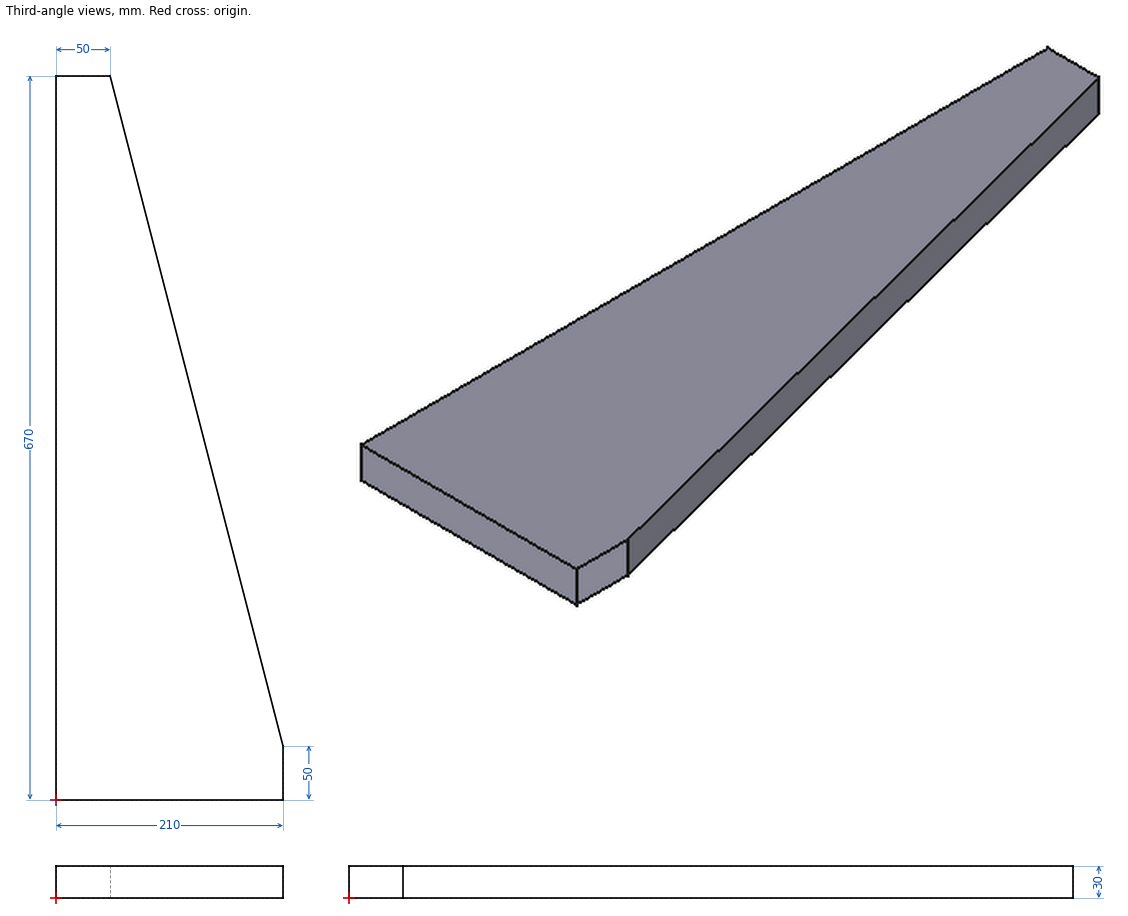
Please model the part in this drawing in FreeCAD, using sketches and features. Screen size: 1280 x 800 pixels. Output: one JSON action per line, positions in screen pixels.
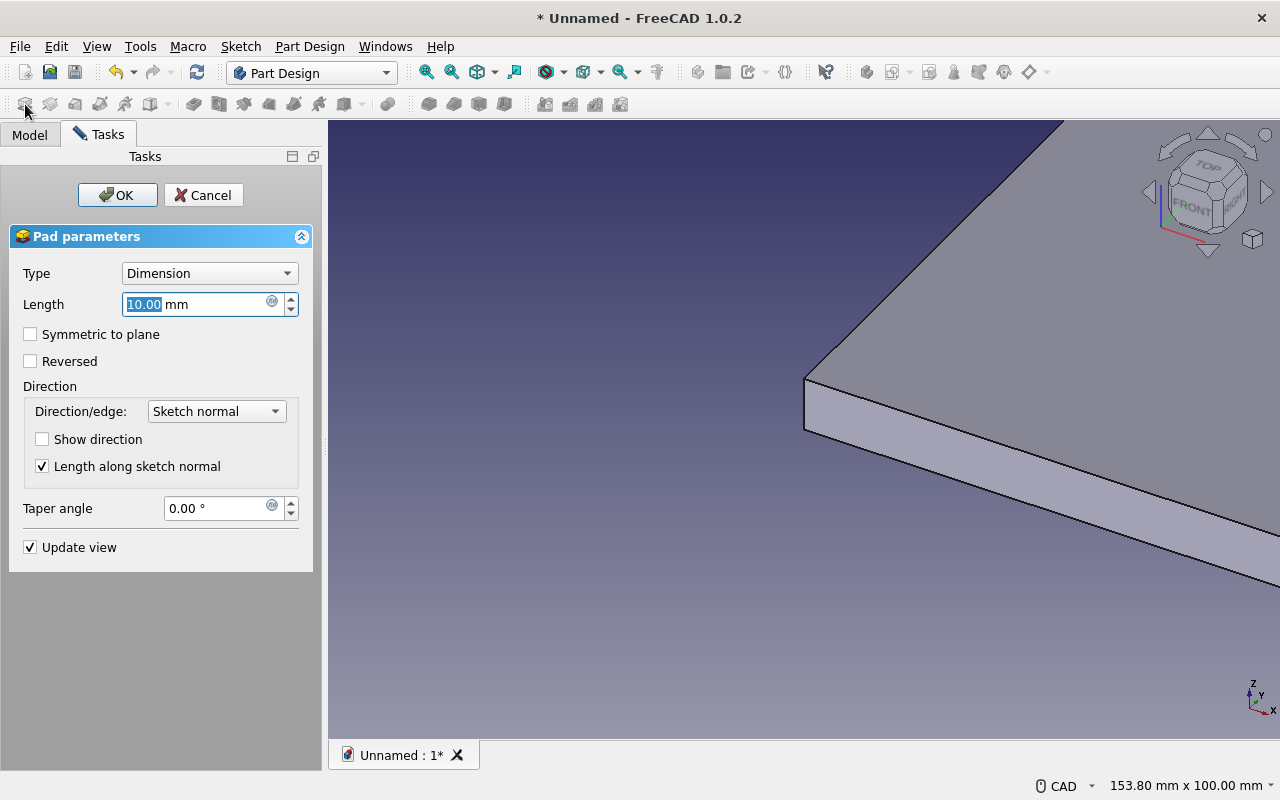
{"action": "type", "text": "30"}
{"action": "key", "text": "Tab"}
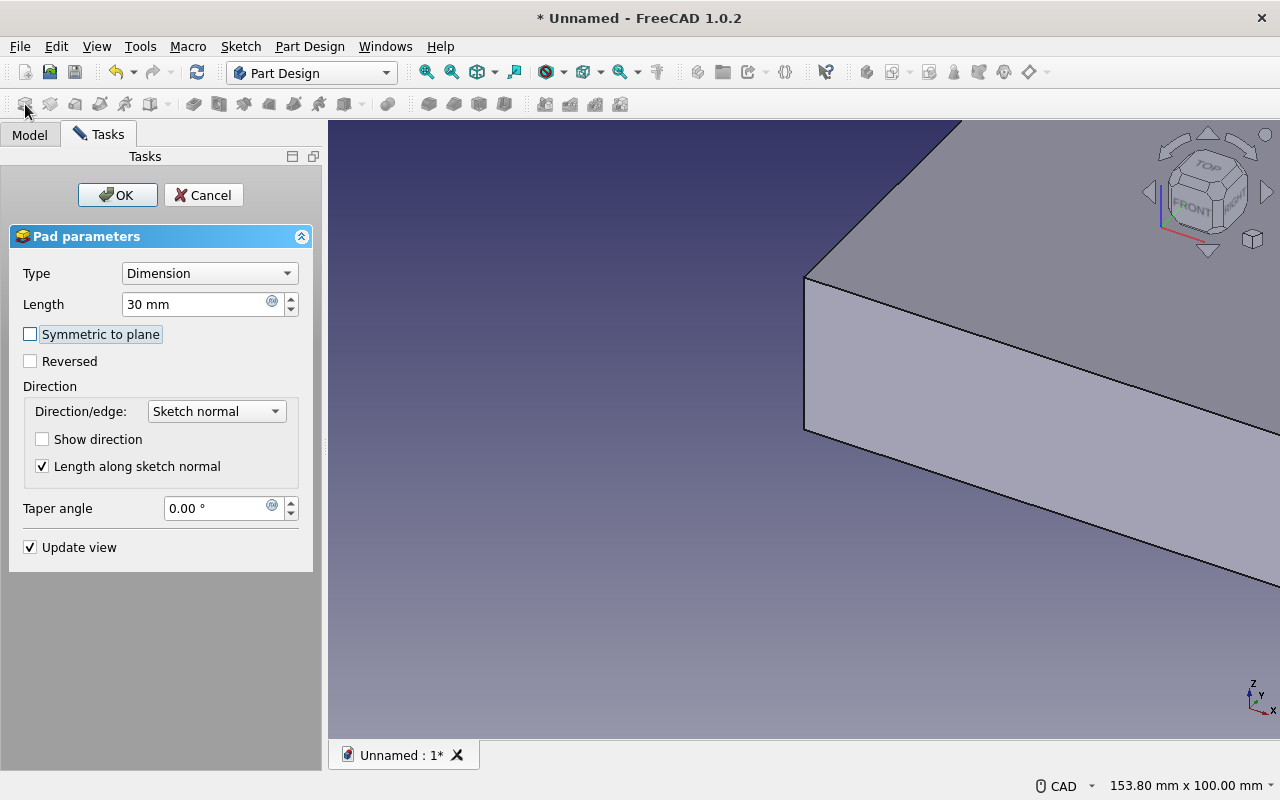
{"action": "left_click", "coordinate": [118, 195]}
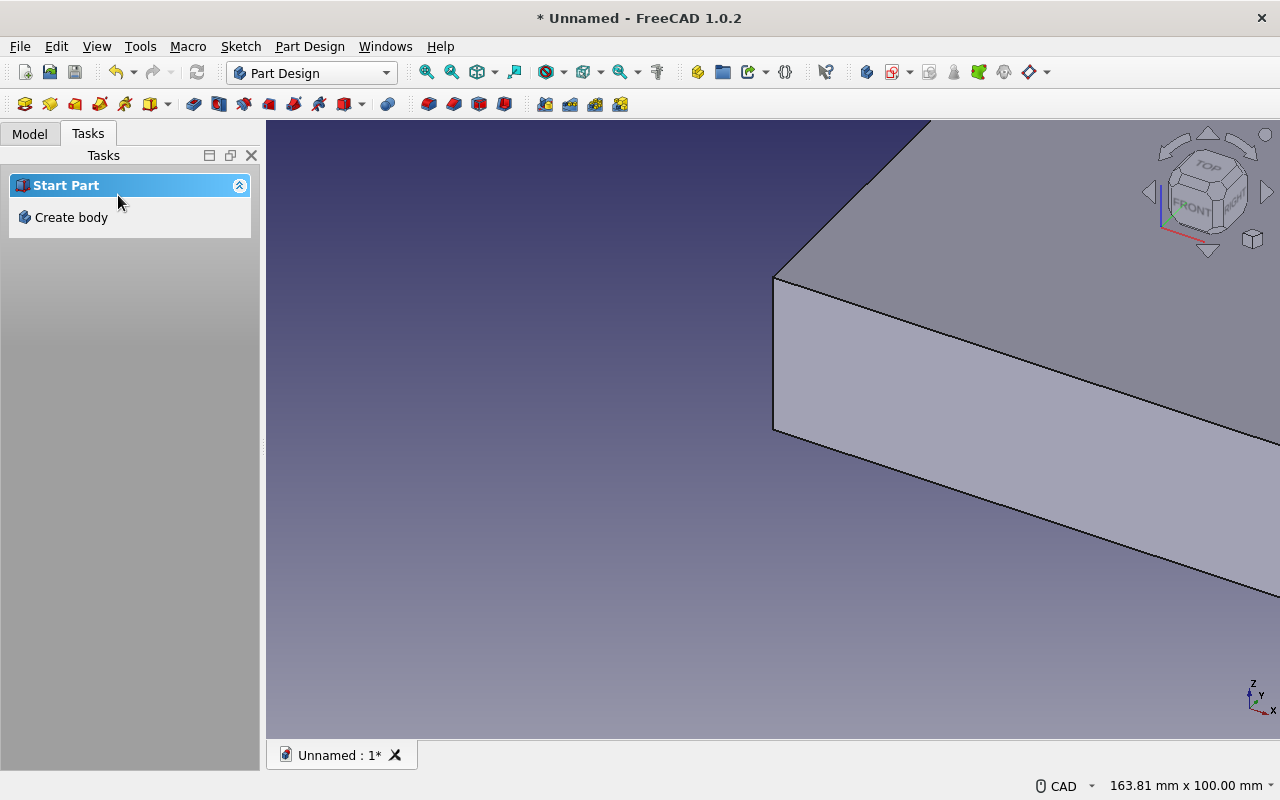
{"action": "key", "text": "0"}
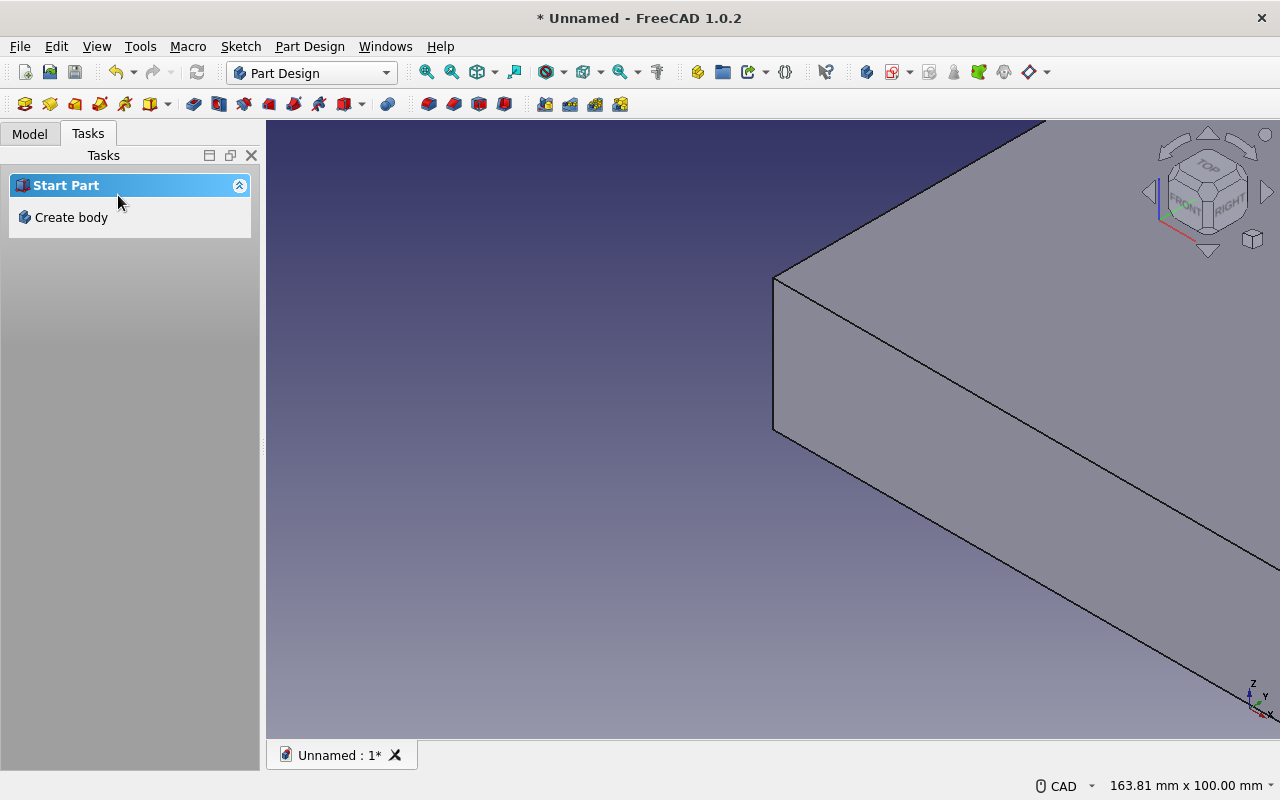
{"action": "left_click", "coordinate": [427, 72]}